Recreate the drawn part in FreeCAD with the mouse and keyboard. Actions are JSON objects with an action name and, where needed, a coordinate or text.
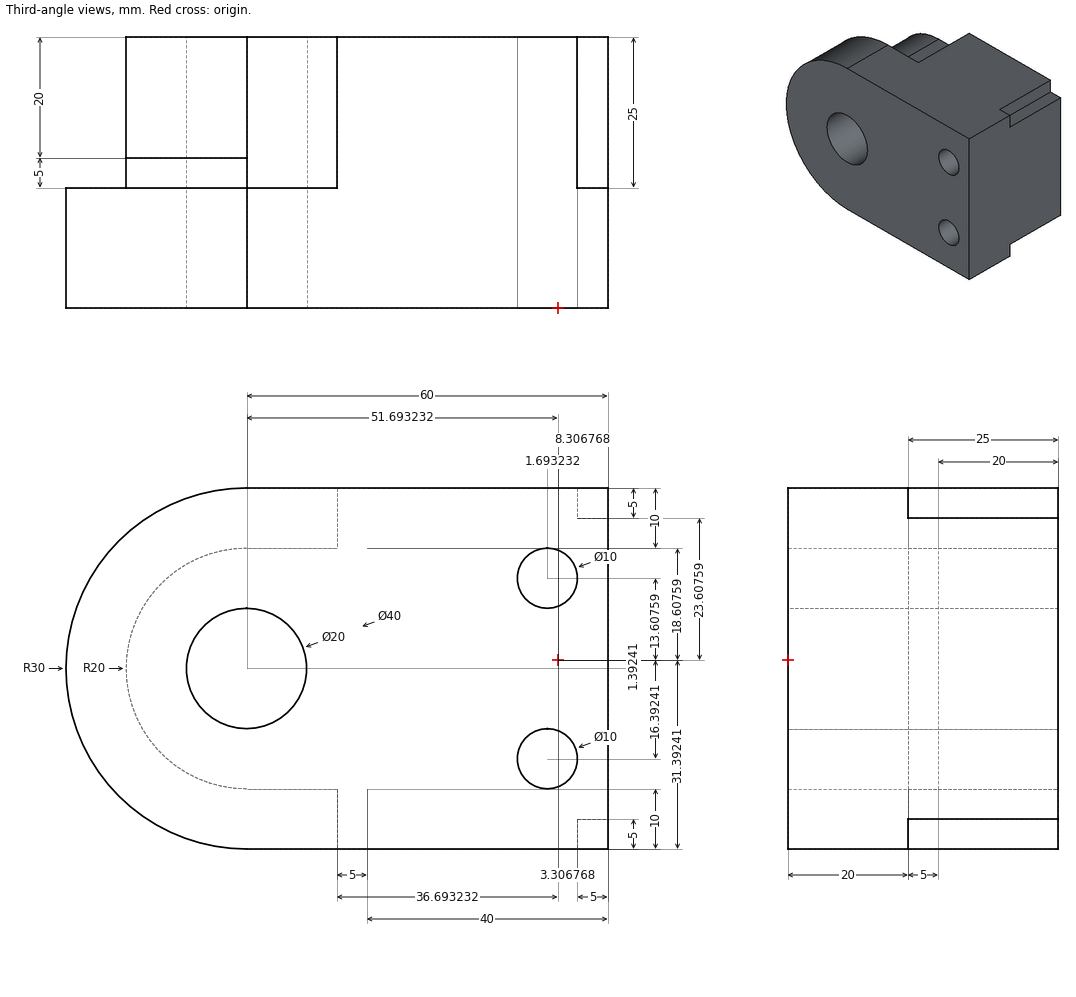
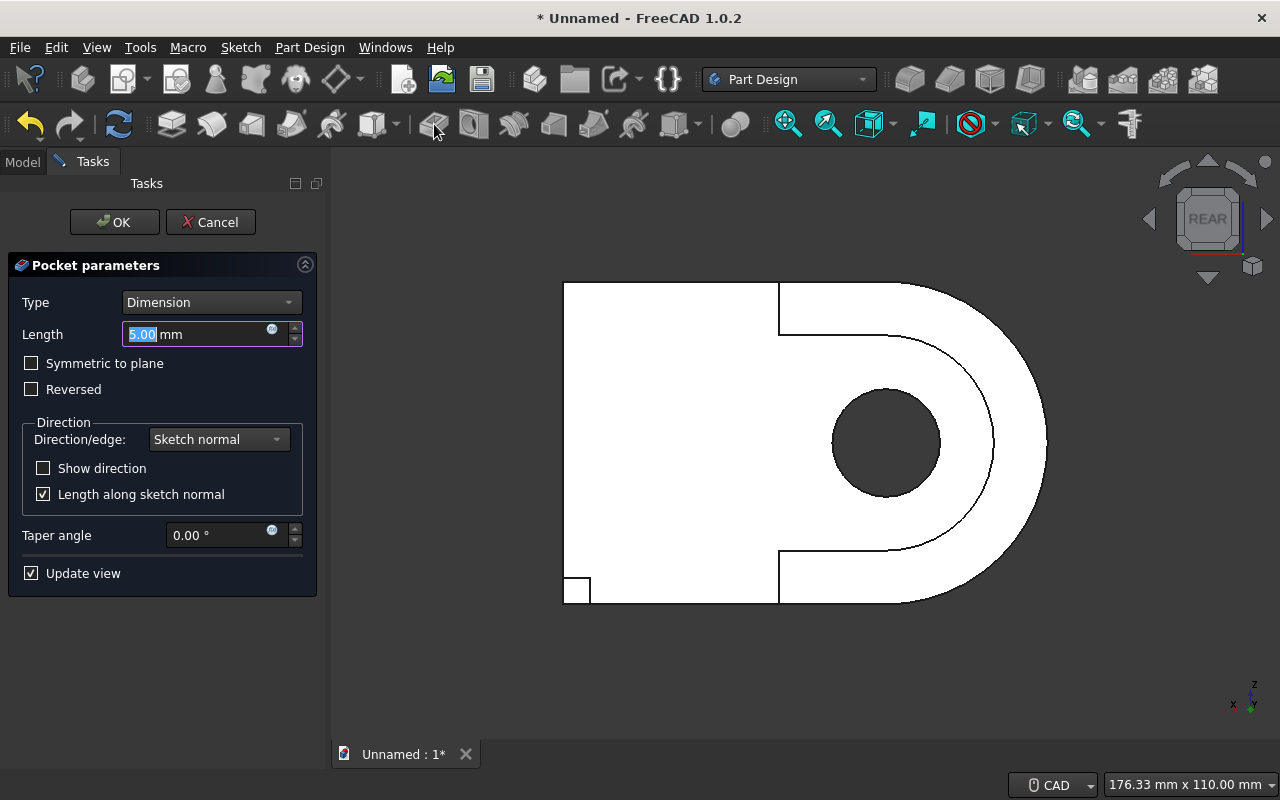
{"action": "type", "text": "25"}
{"action": "key", "text": "Tab"}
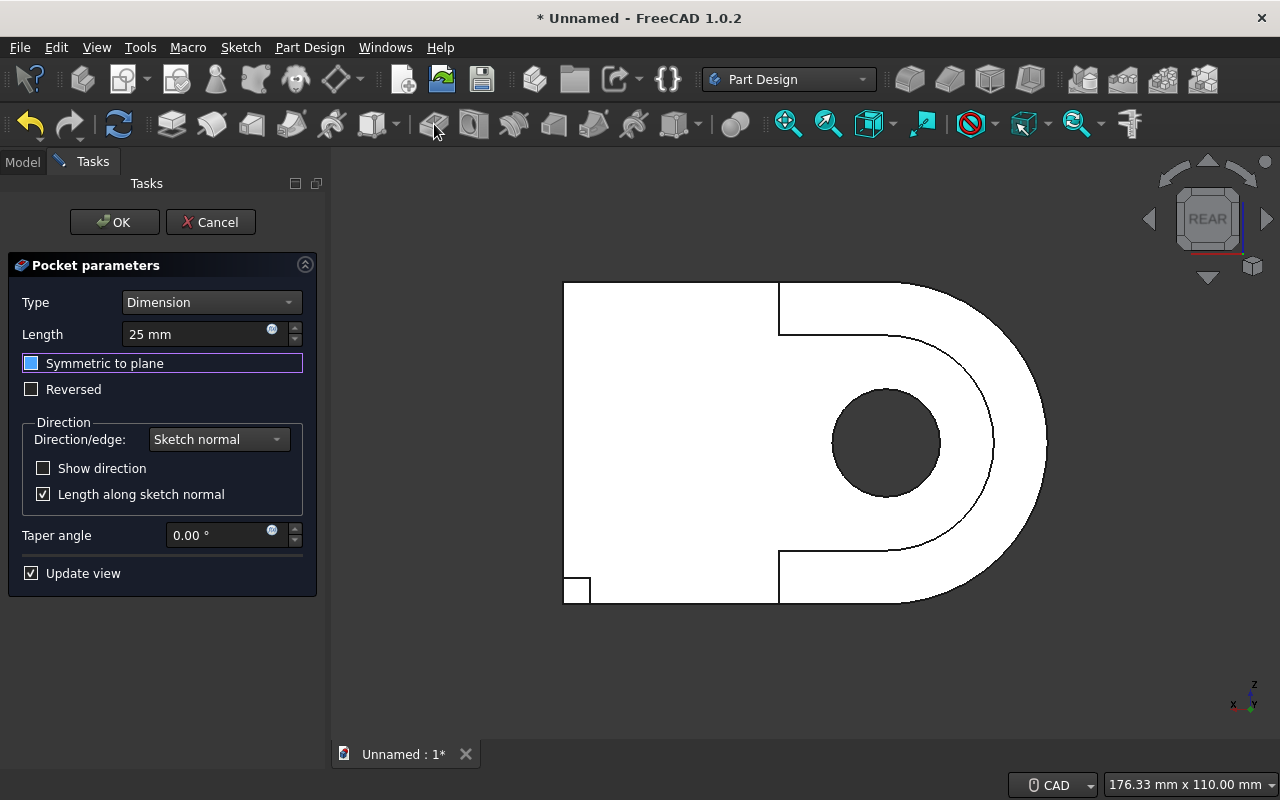
{"action": "left_click", "coordinate": [115, 222]}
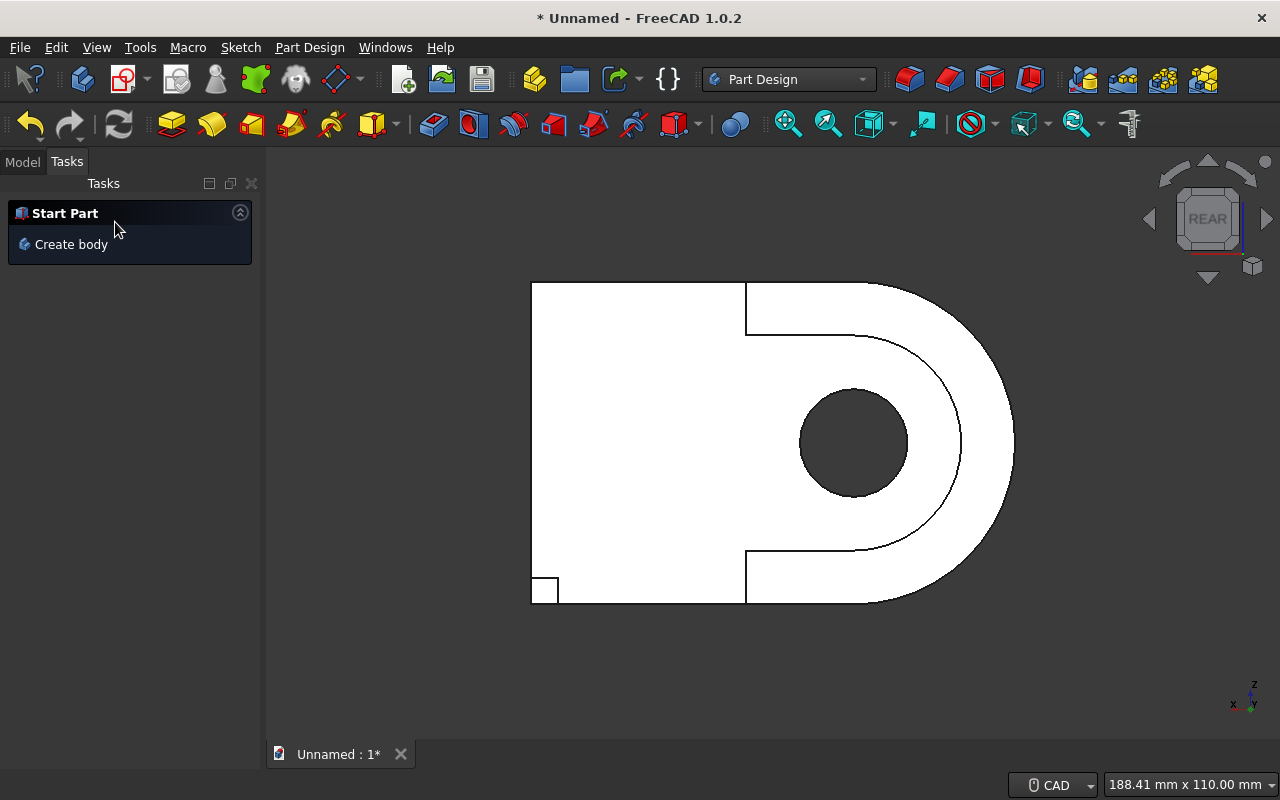
{"action": "left_click", "coordinate": [685, 442]}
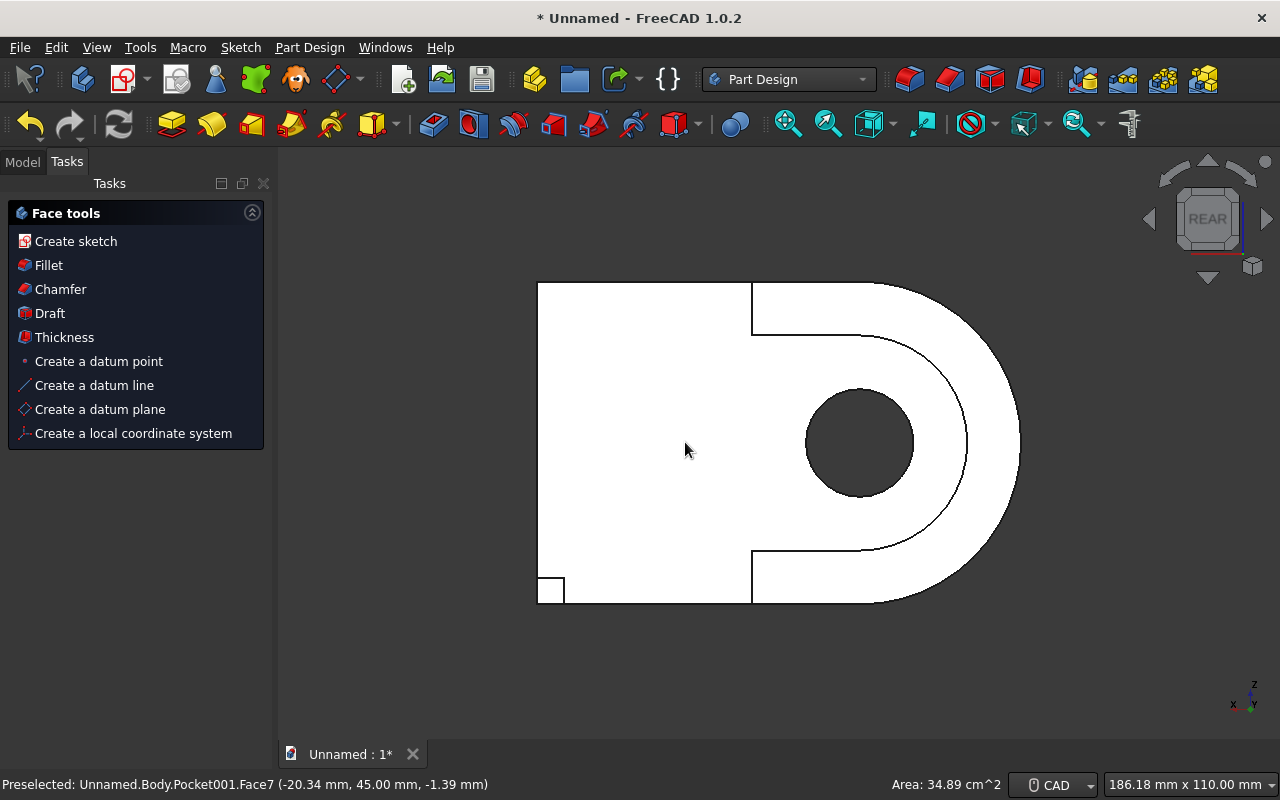
{"action": "left_click", "coordinate": [124, 80]}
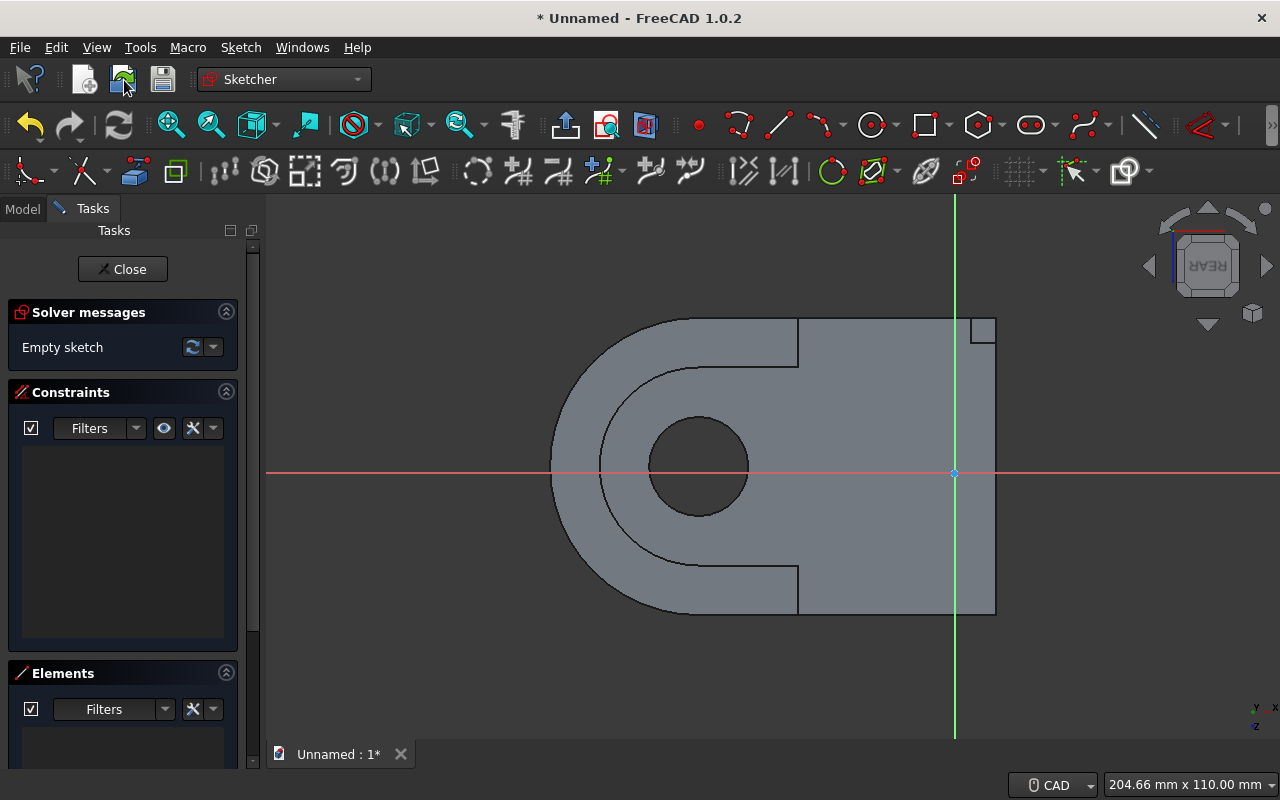
{"action": "scroll", "coordinate": [1006, 614], "scroll_direction": "up", "scroll_amount": 13}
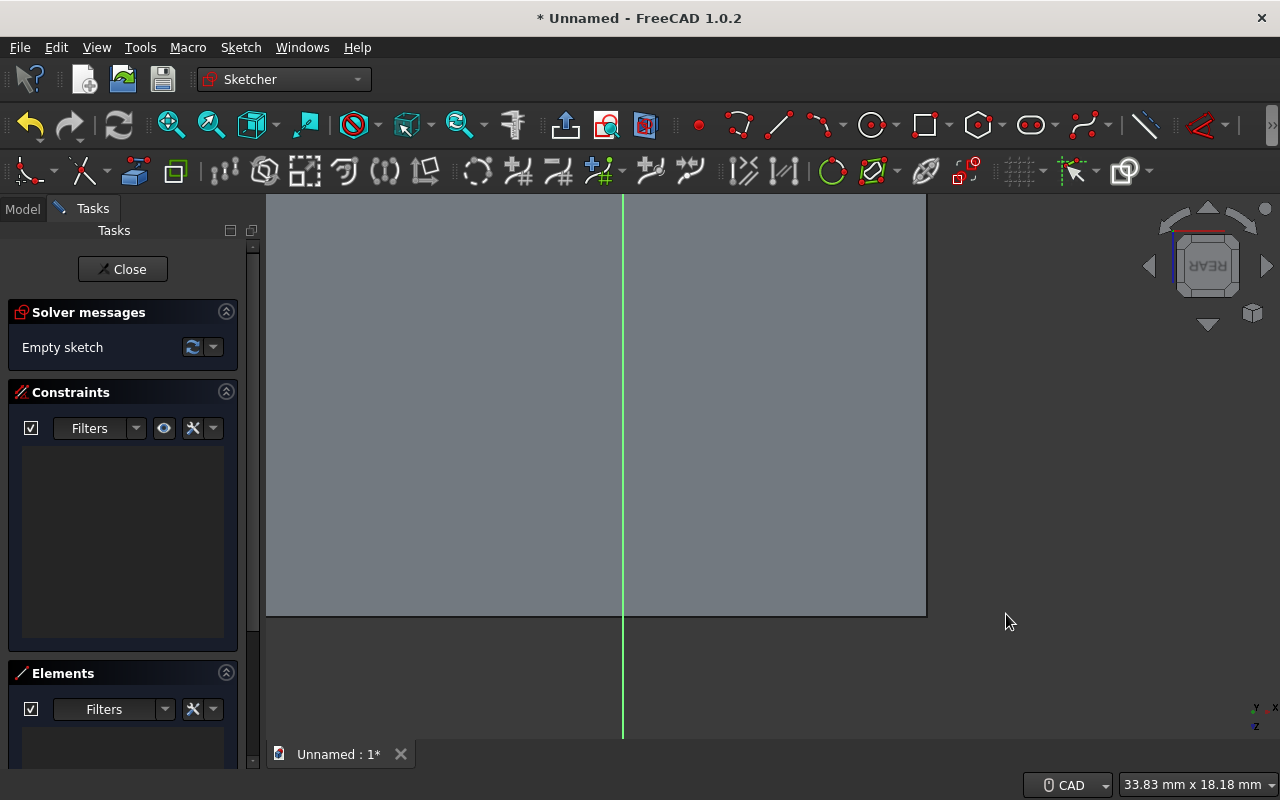
{"action": "key", "text": "g r"}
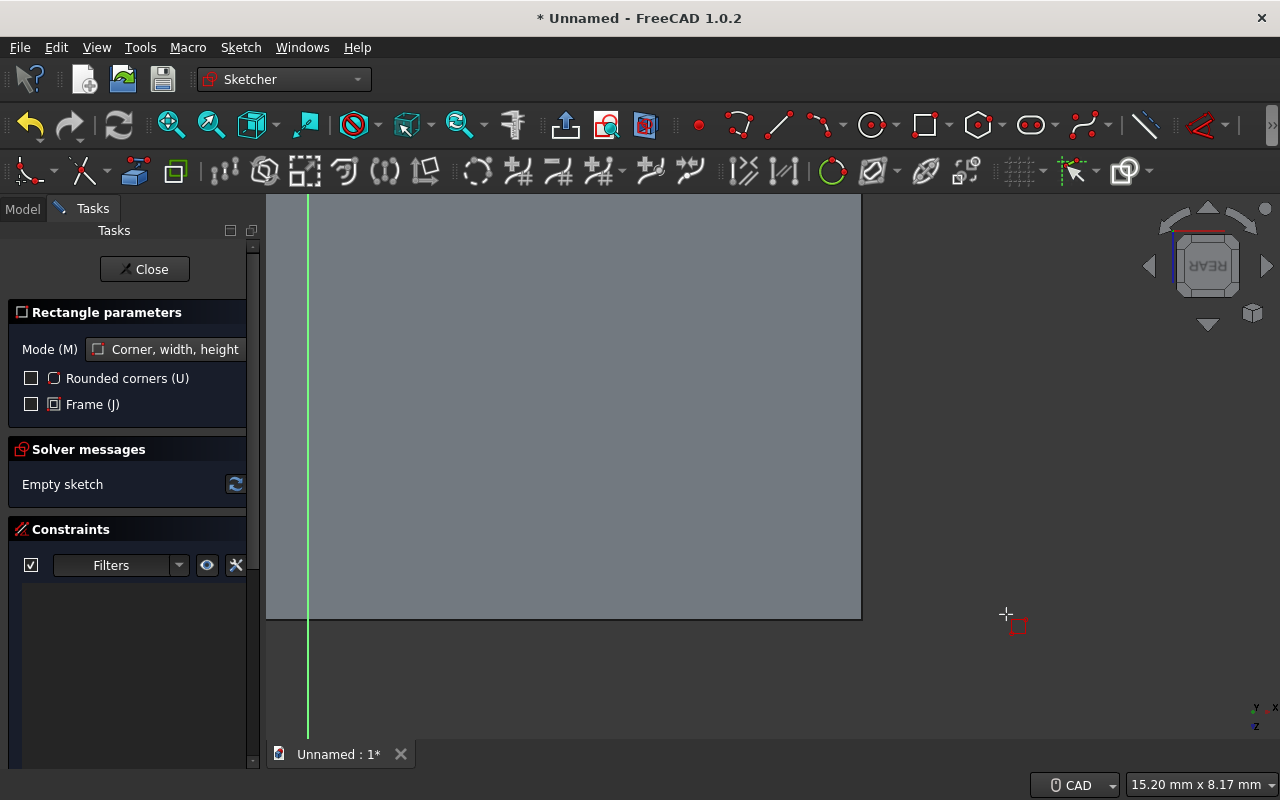
{"action": "left_click", "coordinate": [528, 286]}
{"action": "left_click", "coordinate": [862, 620]}
{"action": "key", "text": "Escape"}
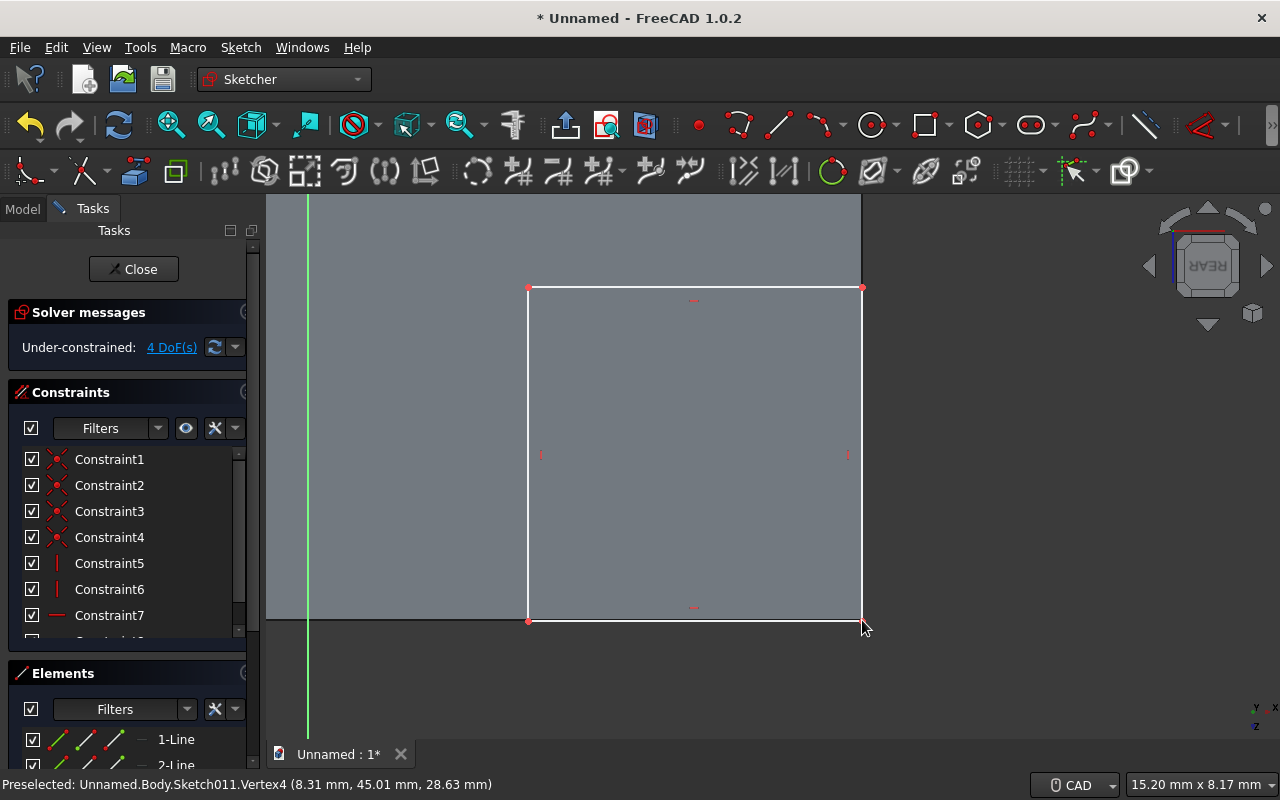
{"action": "key", "text": "d"}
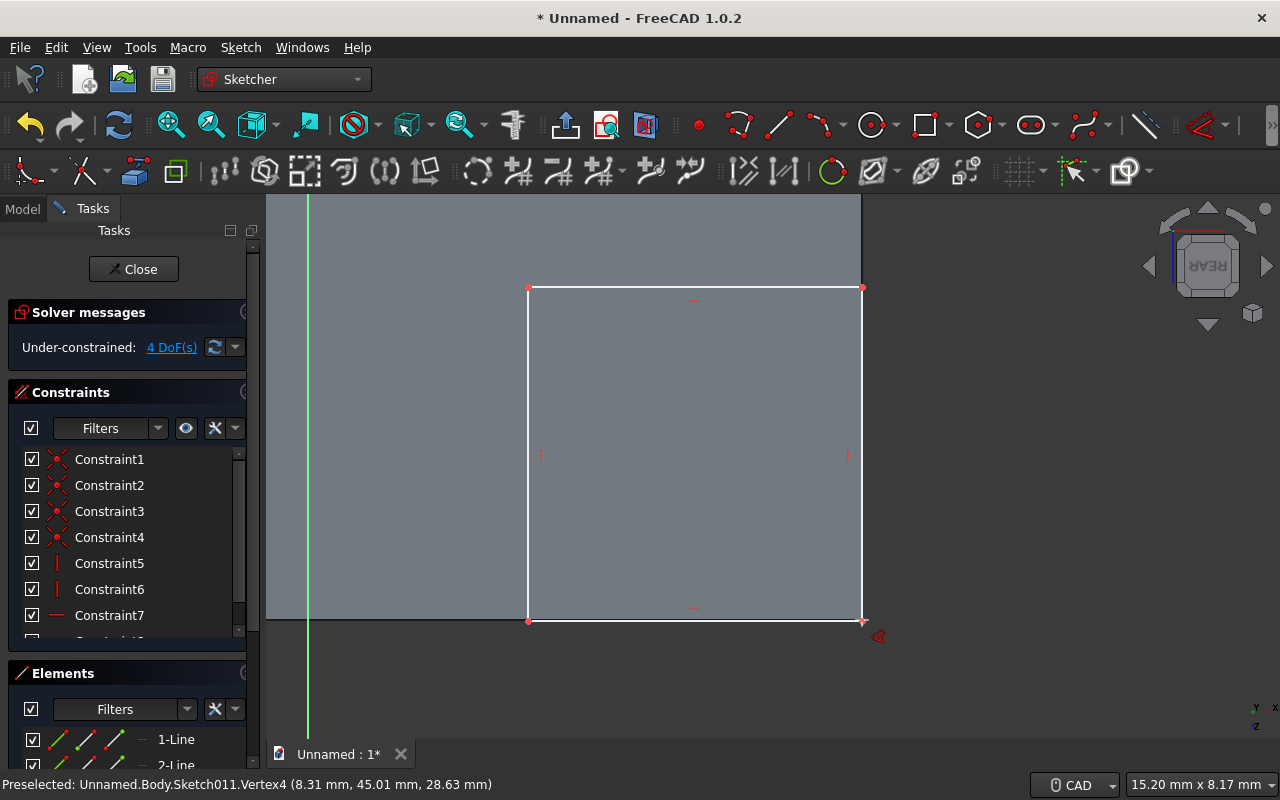
{"action": "left_click", "coordinate": [528, 387]}
{"action": "left_click", "coordinate": [494, 454]}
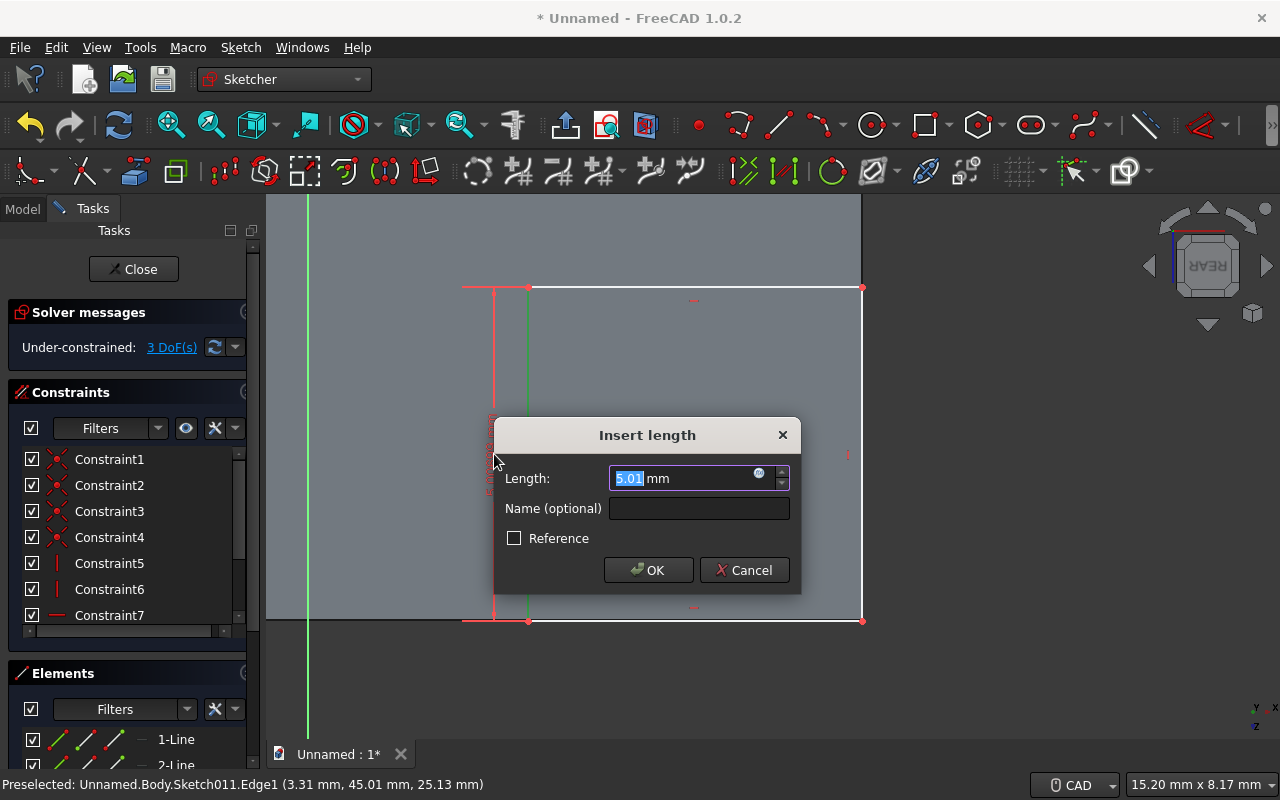
{"action": "type", "text": "5"}
{"action": "key", "text": "Return"}